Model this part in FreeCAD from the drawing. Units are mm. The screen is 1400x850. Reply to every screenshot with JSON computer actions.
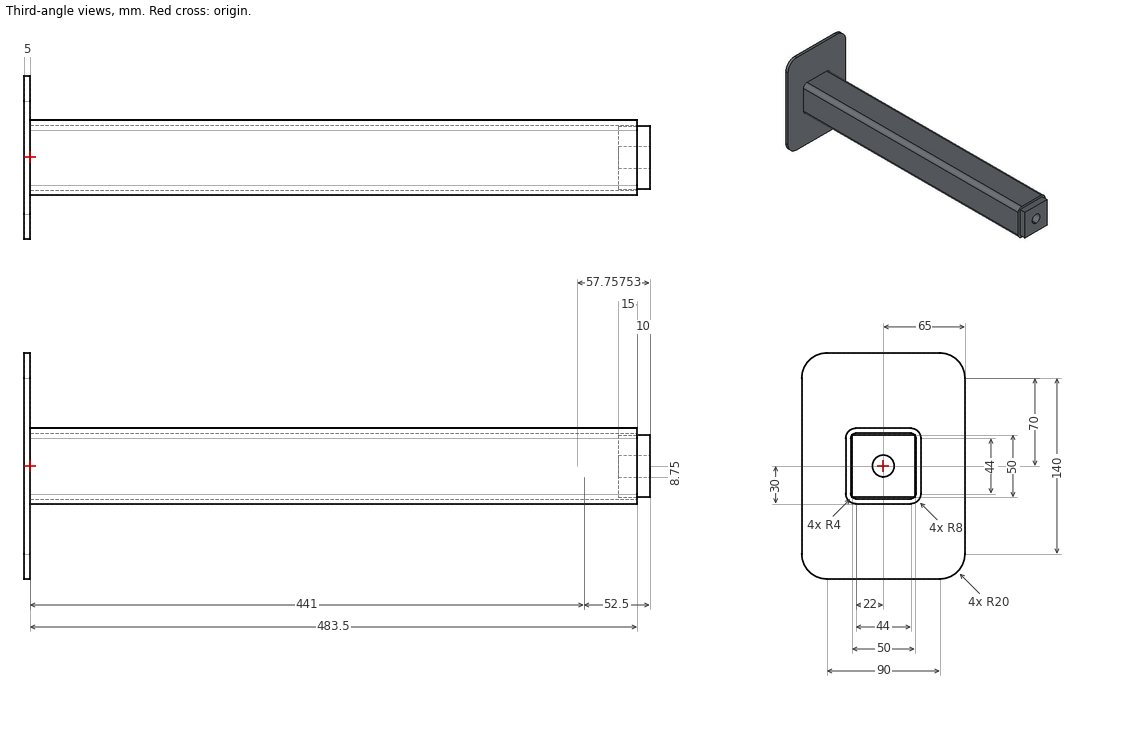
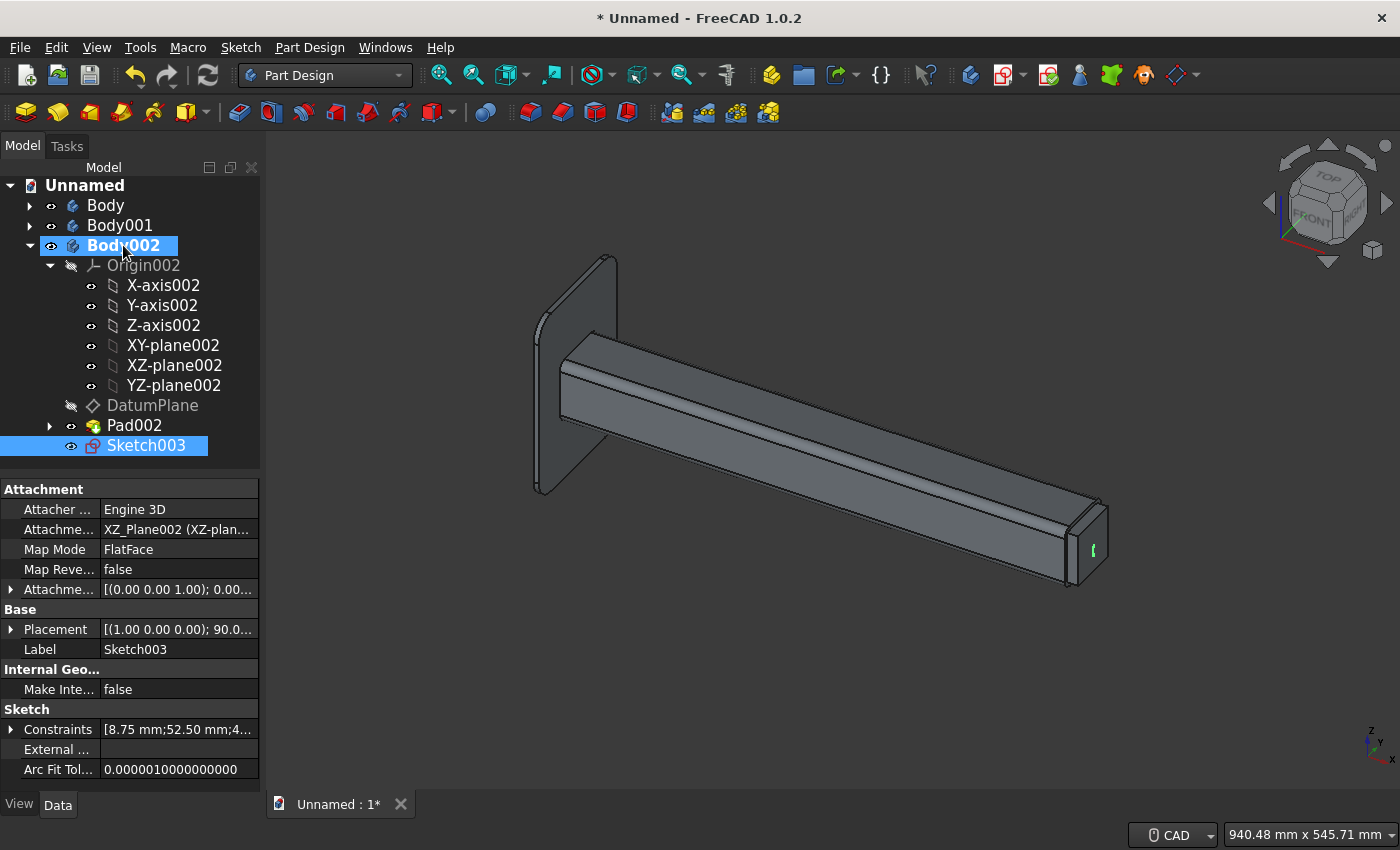
{"action": "left_click", "coordinate": [304, 112]}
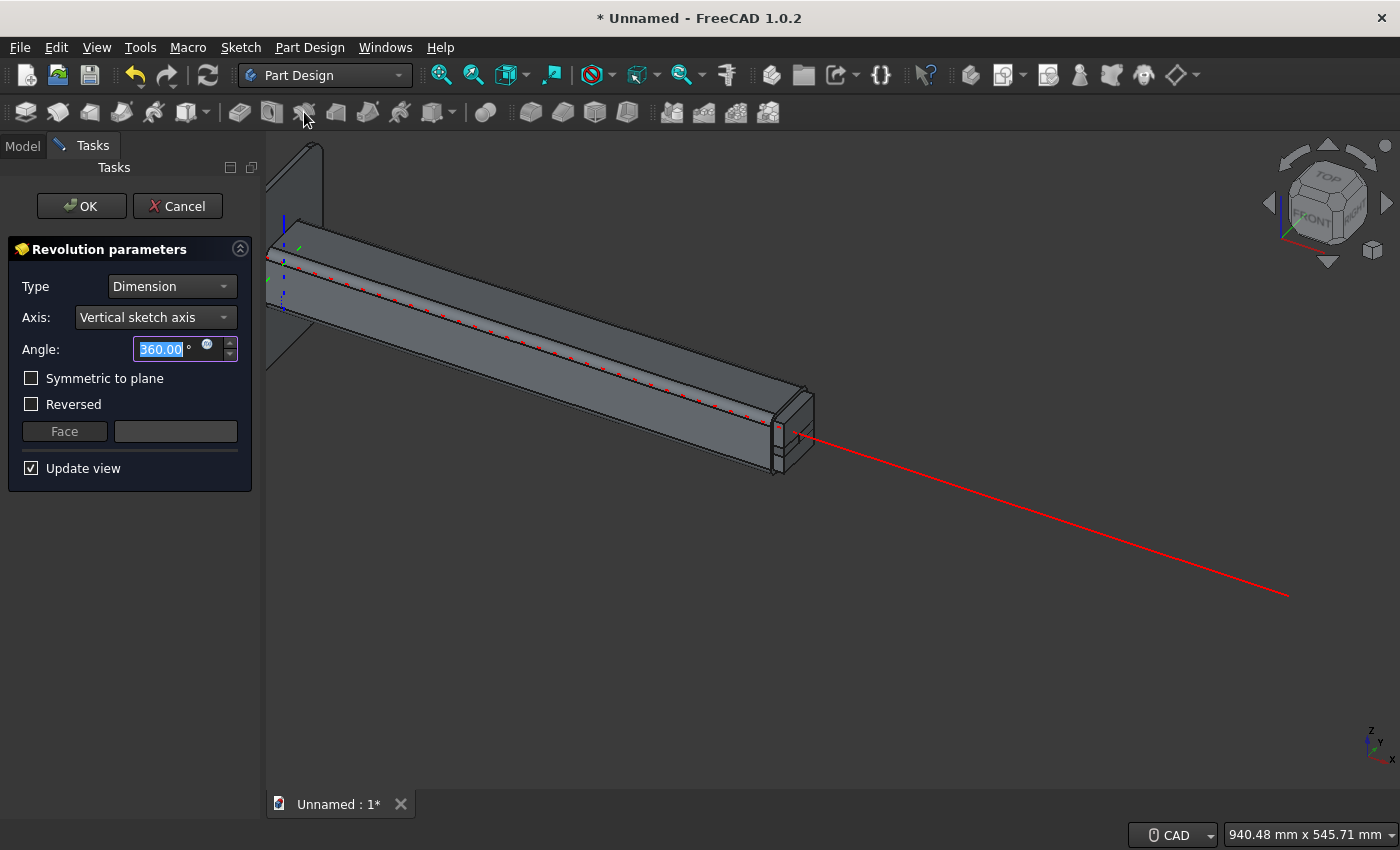
{"action": "left_click", "coordinate": [156, 318]}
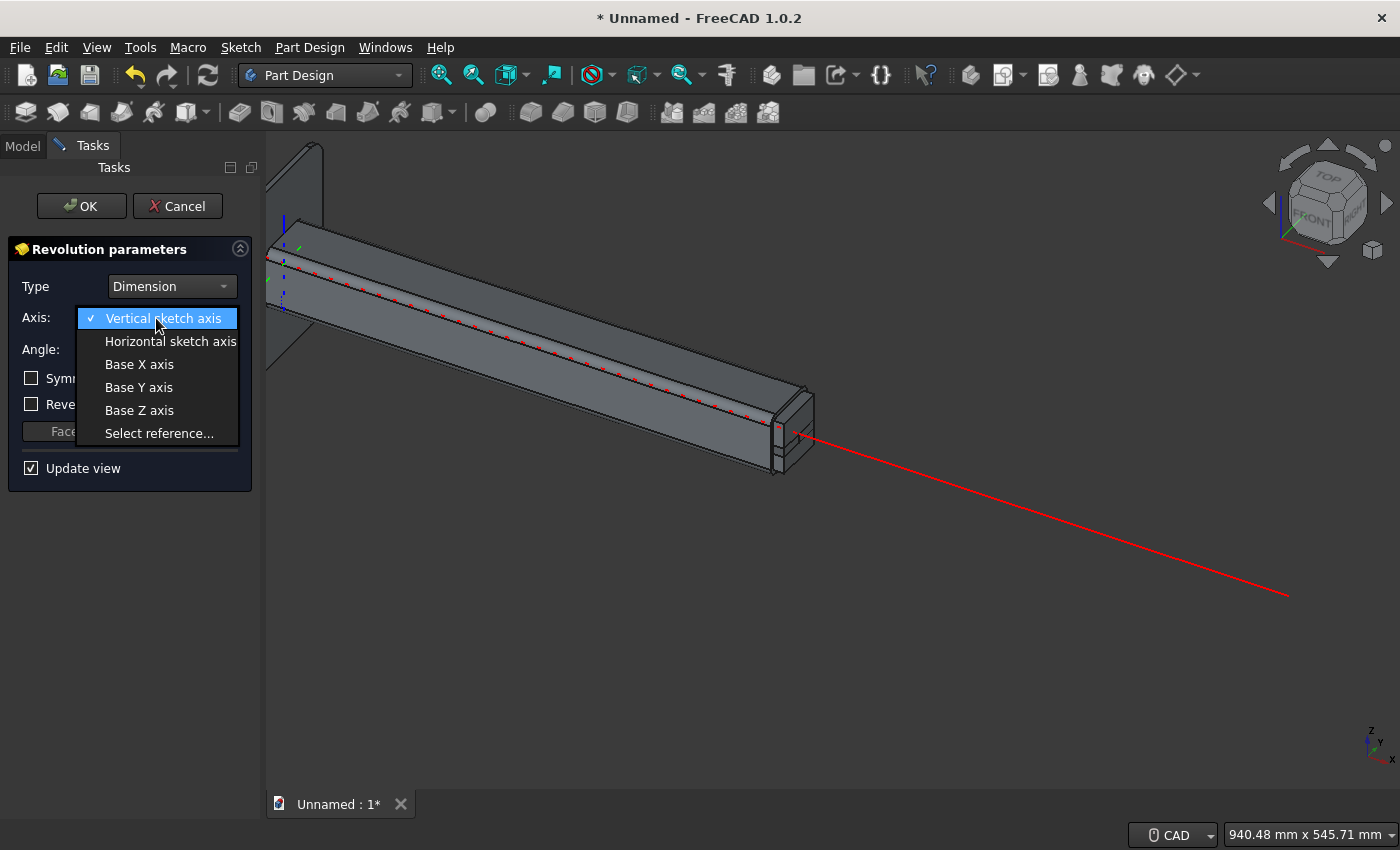
{"action": "left_click", "coordinate": [156, 342]}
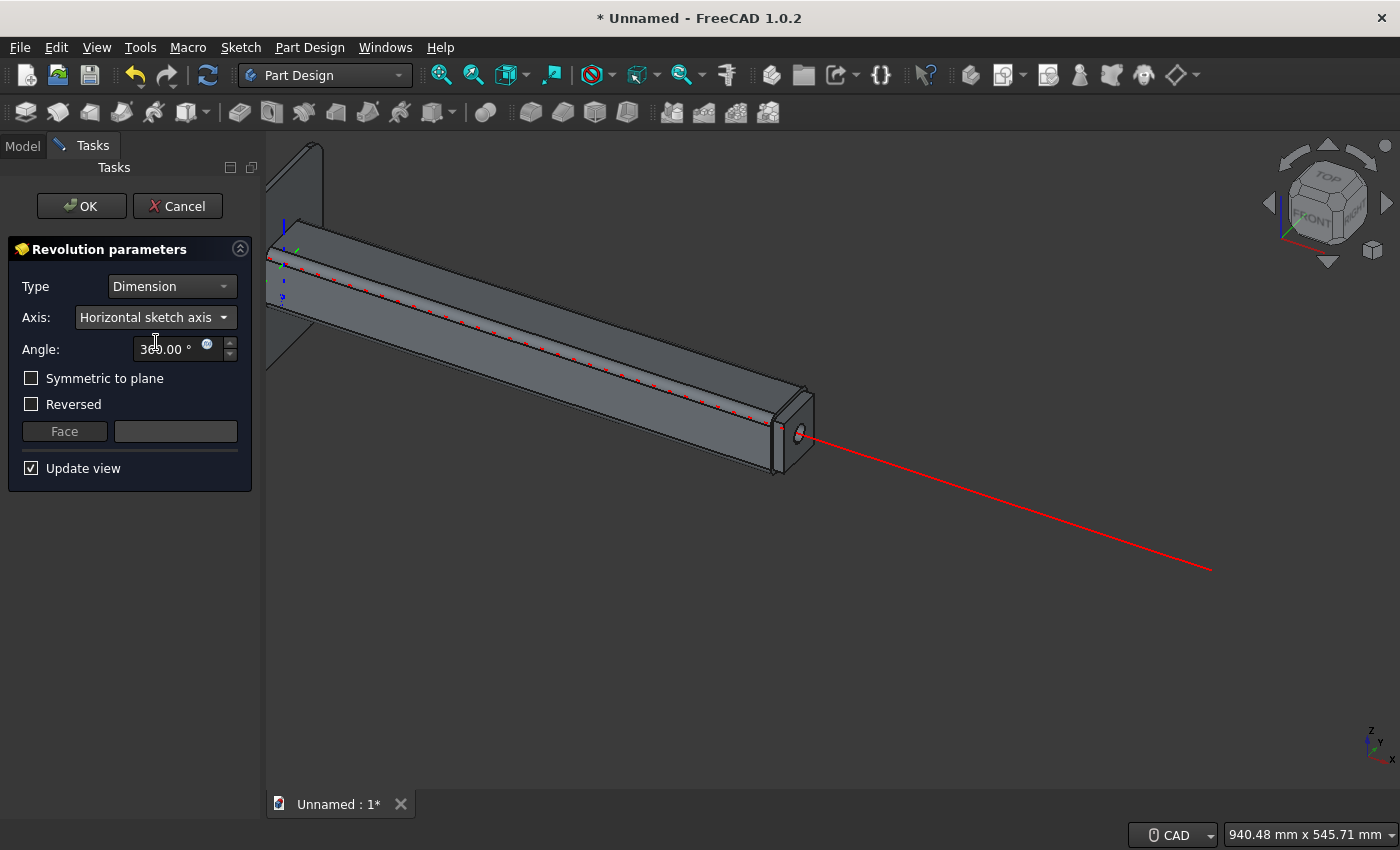
{"action": "left_click", "coordinate": [82, 206]}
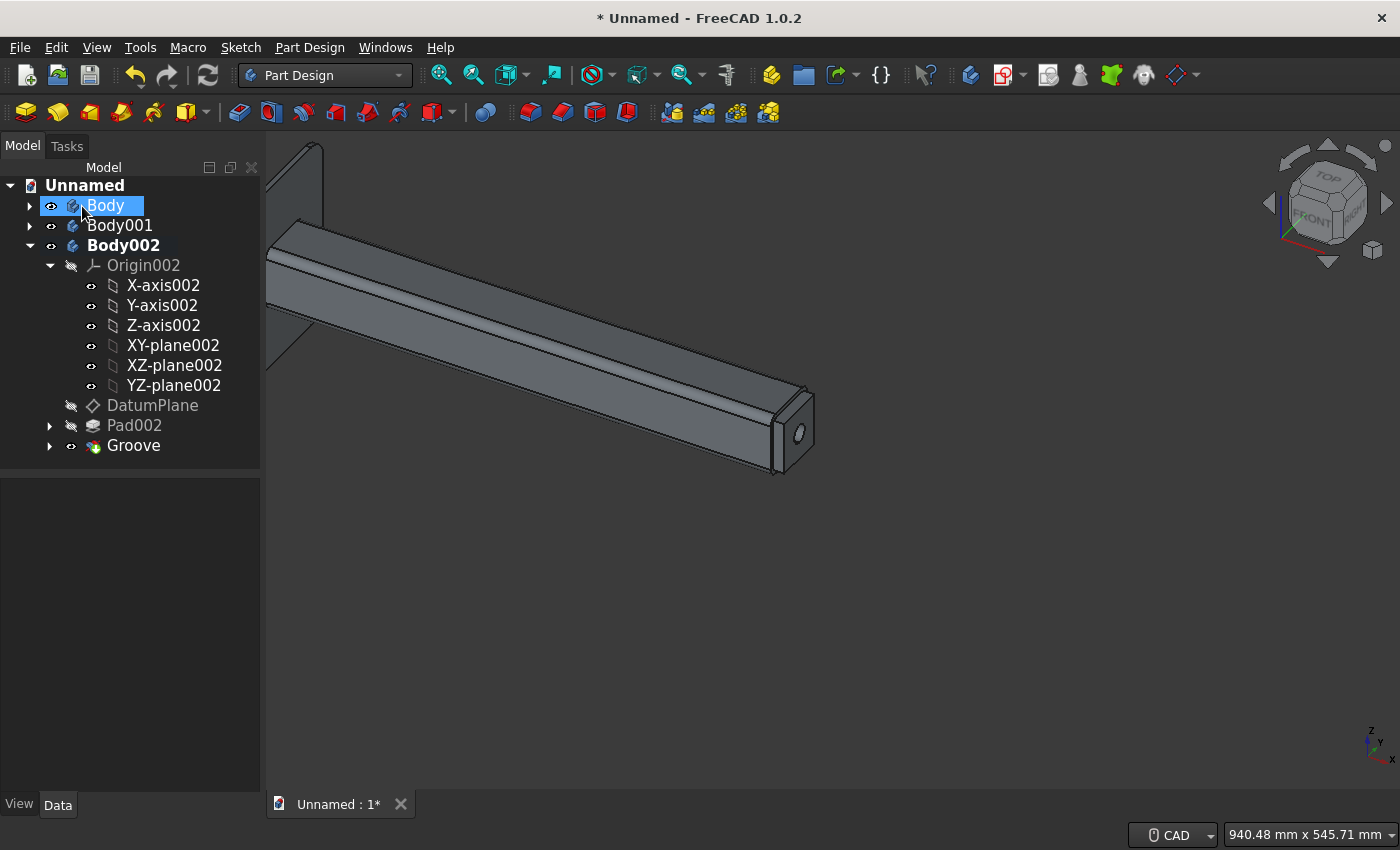
{"action": "key", "text": "0"}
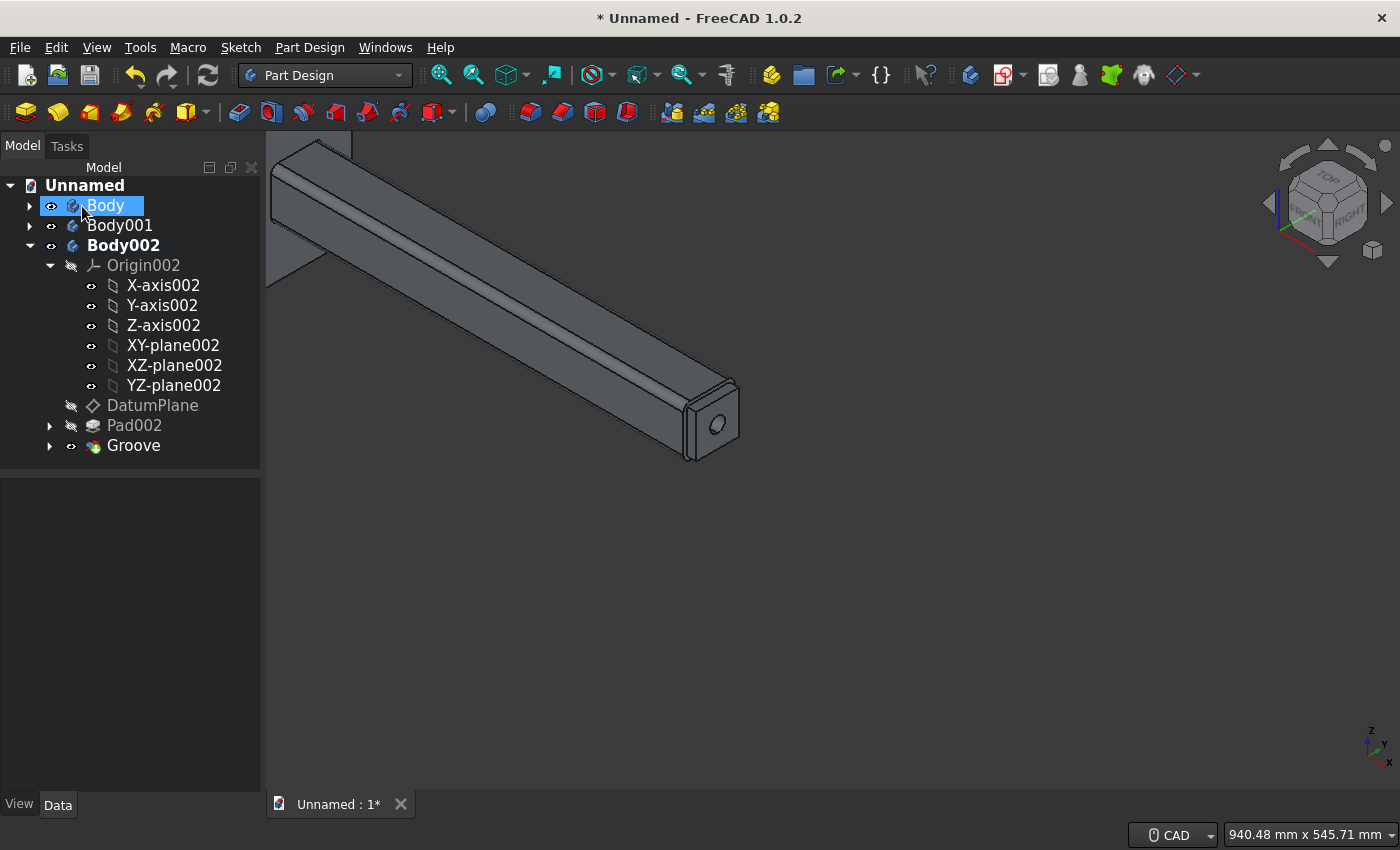
{"action": "left_click", "coordinate": [442, 76]}